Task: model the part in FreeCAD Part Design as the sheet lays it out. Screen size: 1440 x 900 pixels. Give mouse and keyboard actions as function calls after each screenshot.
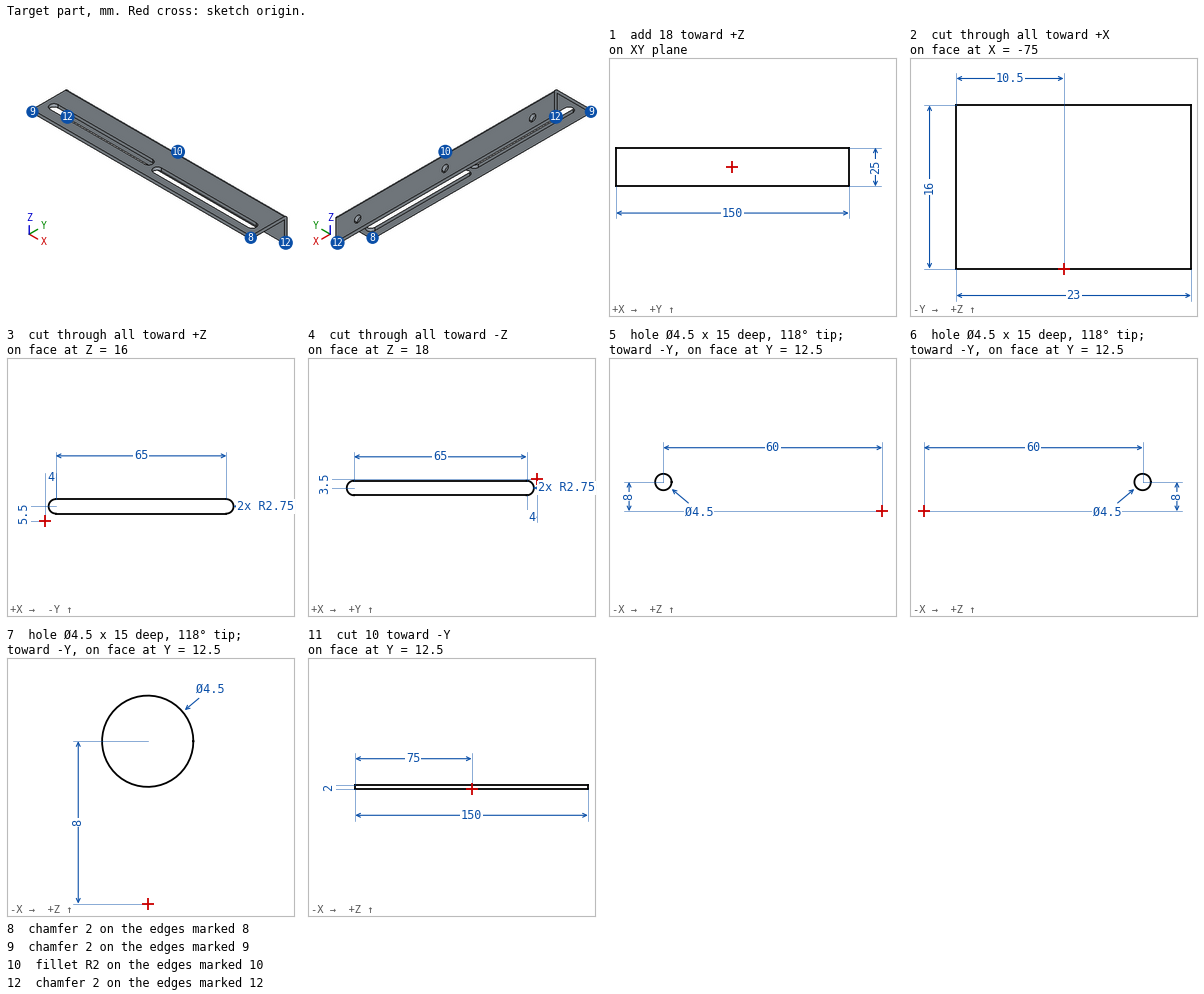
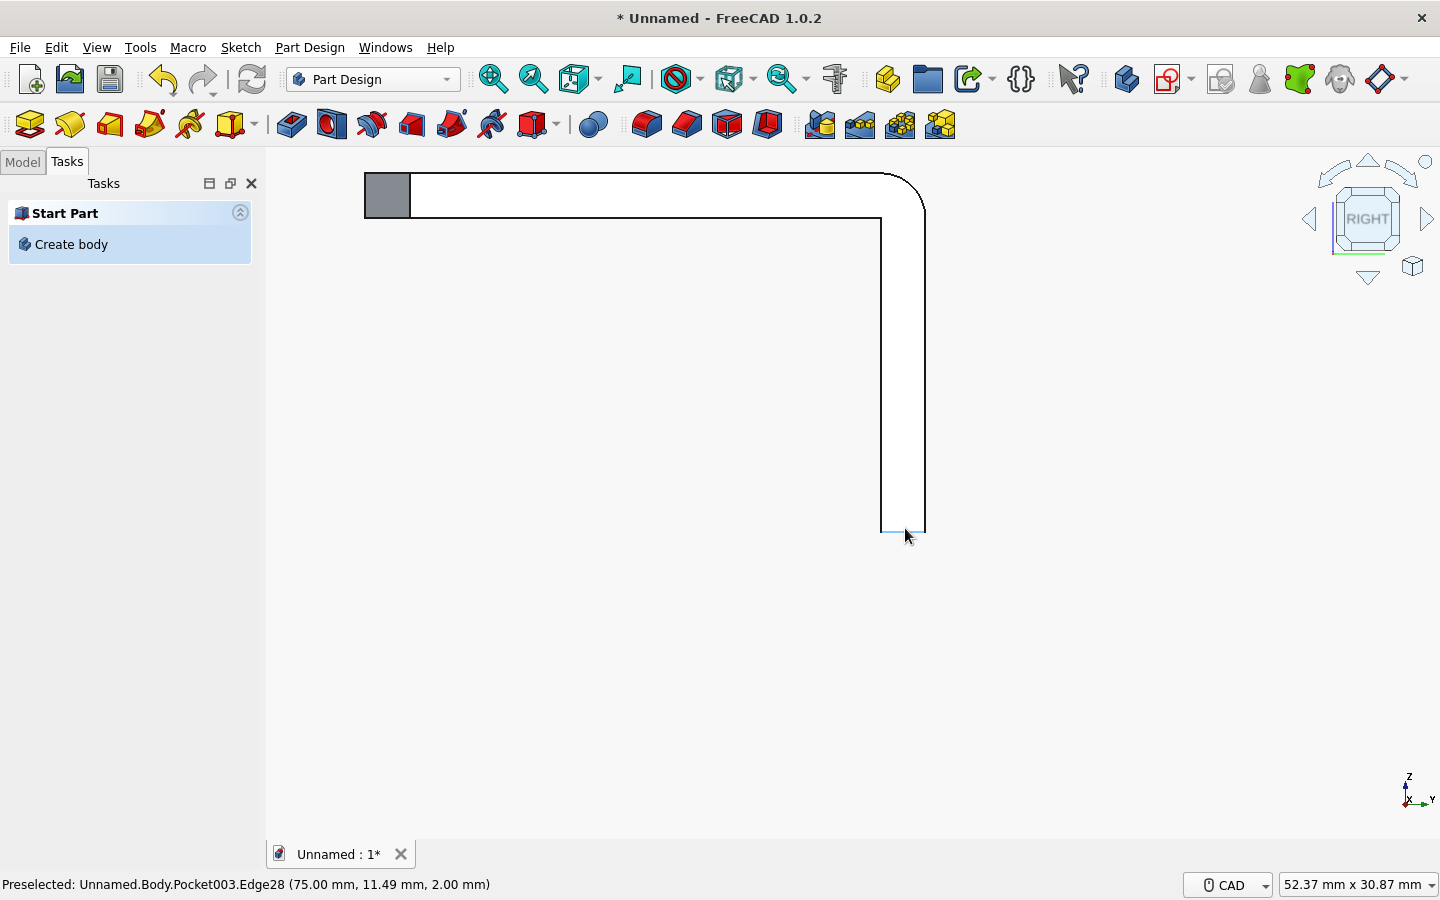
click(903, 531)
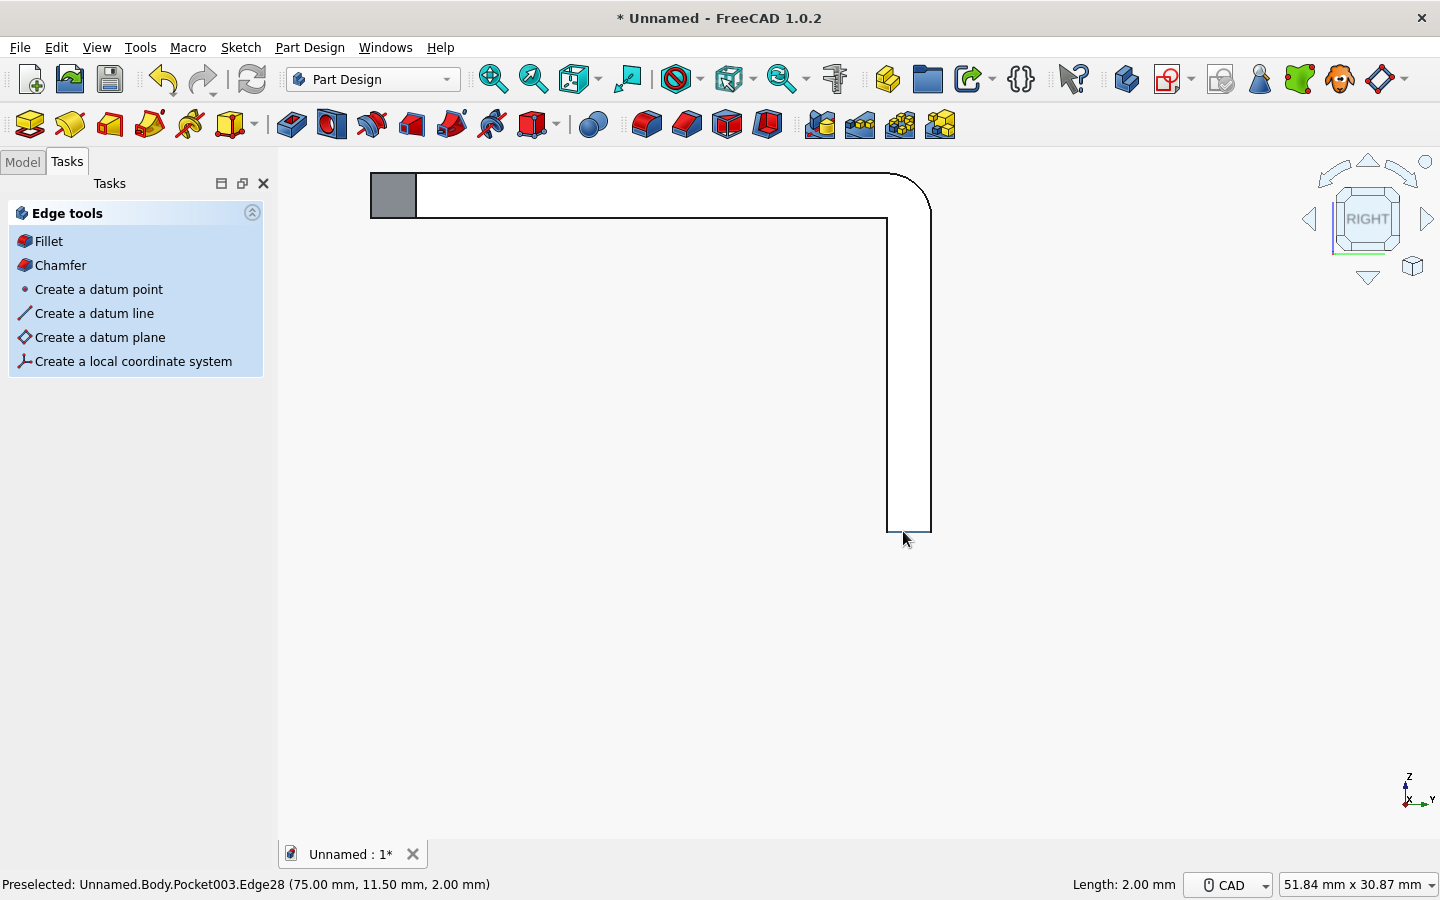
click(494, 80)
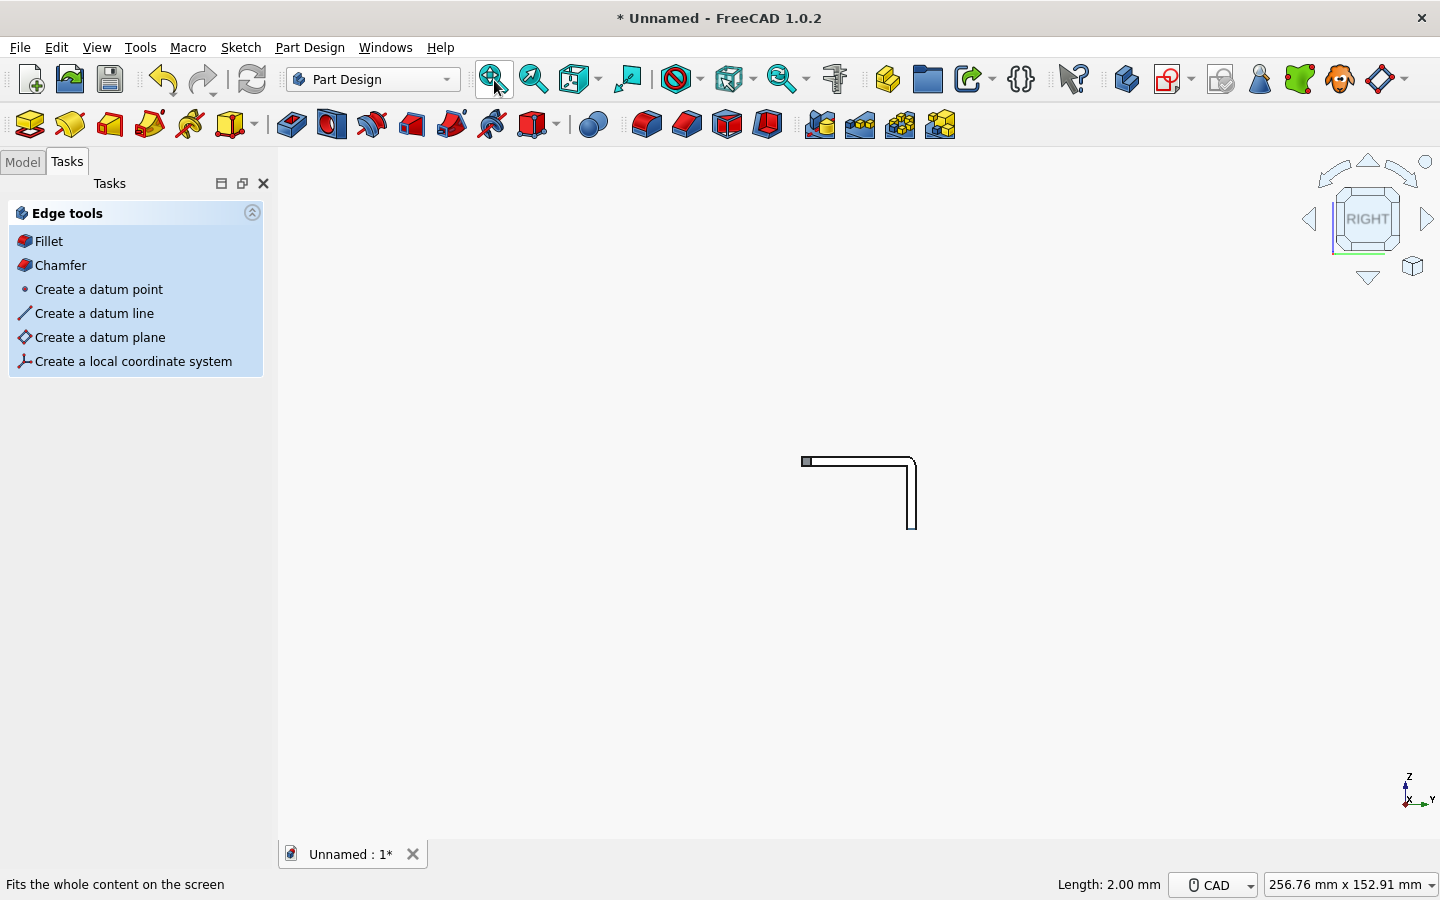
key(5)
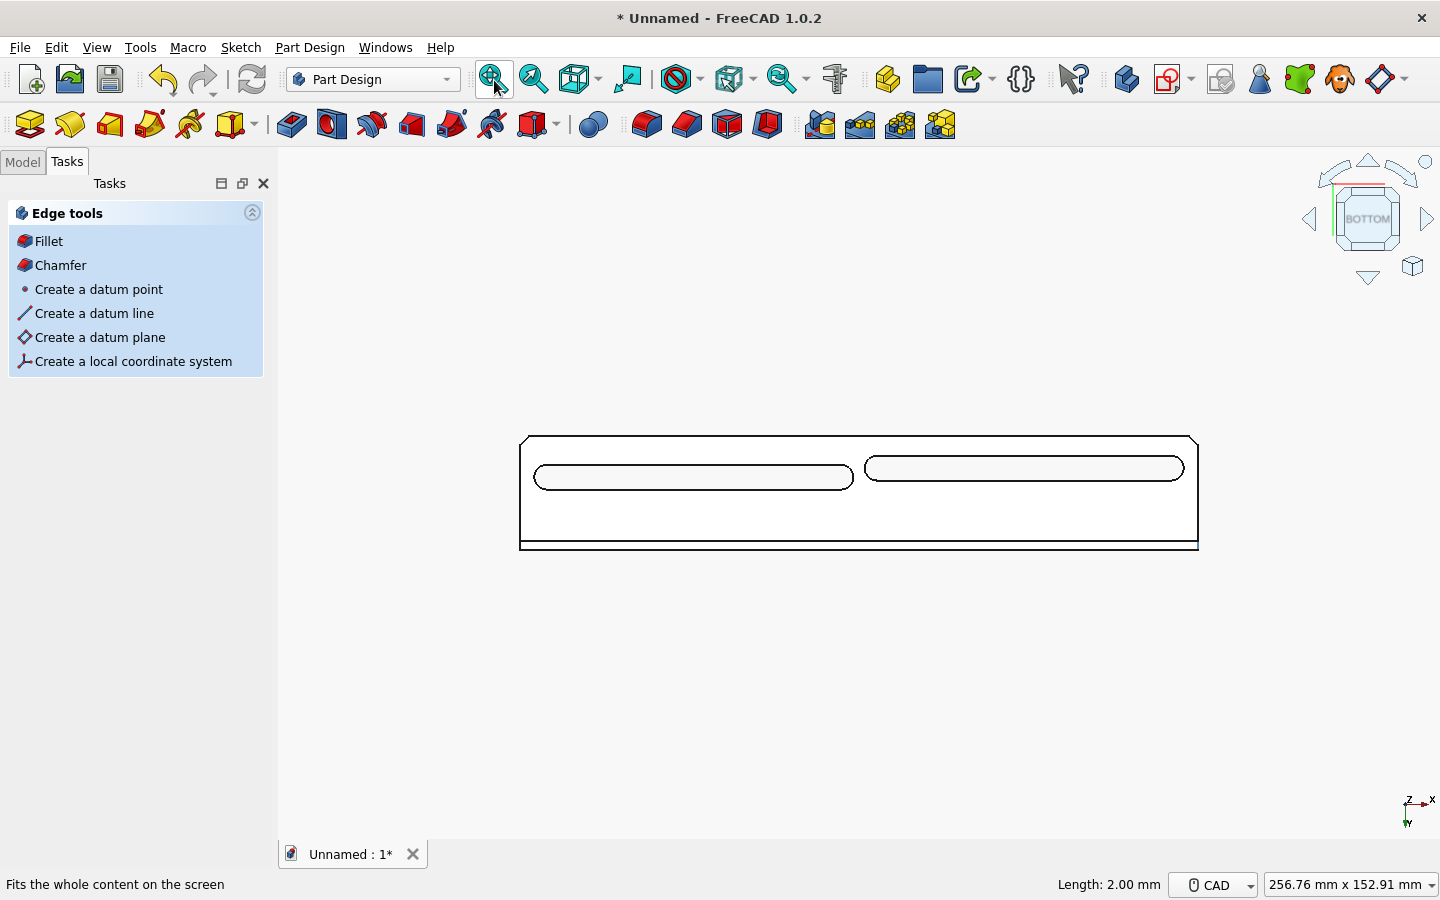
scroll(520, 544, up, 8)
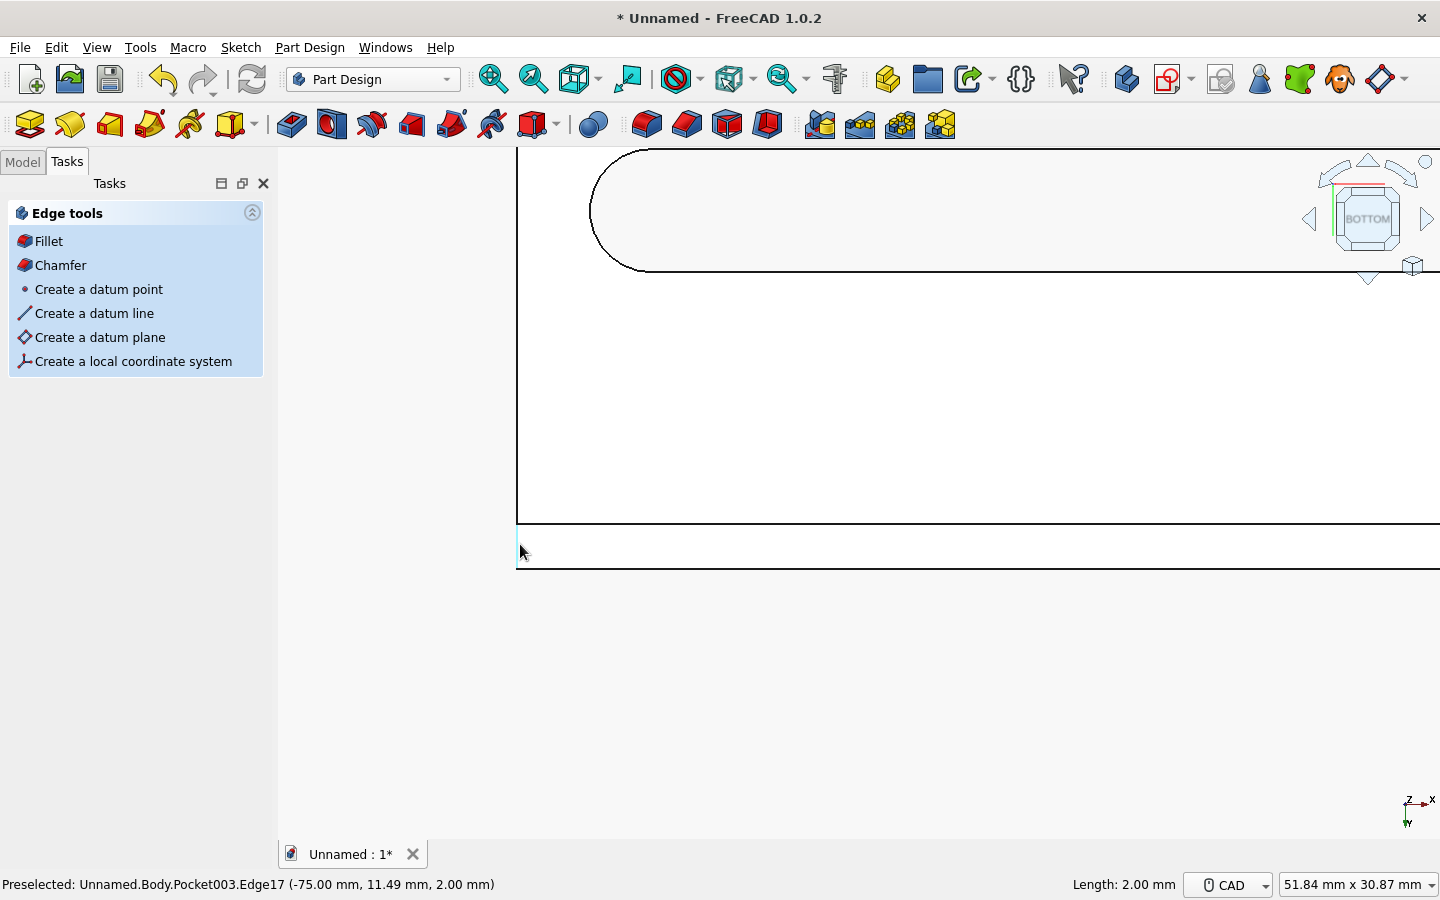
click(517, 546, ctrl)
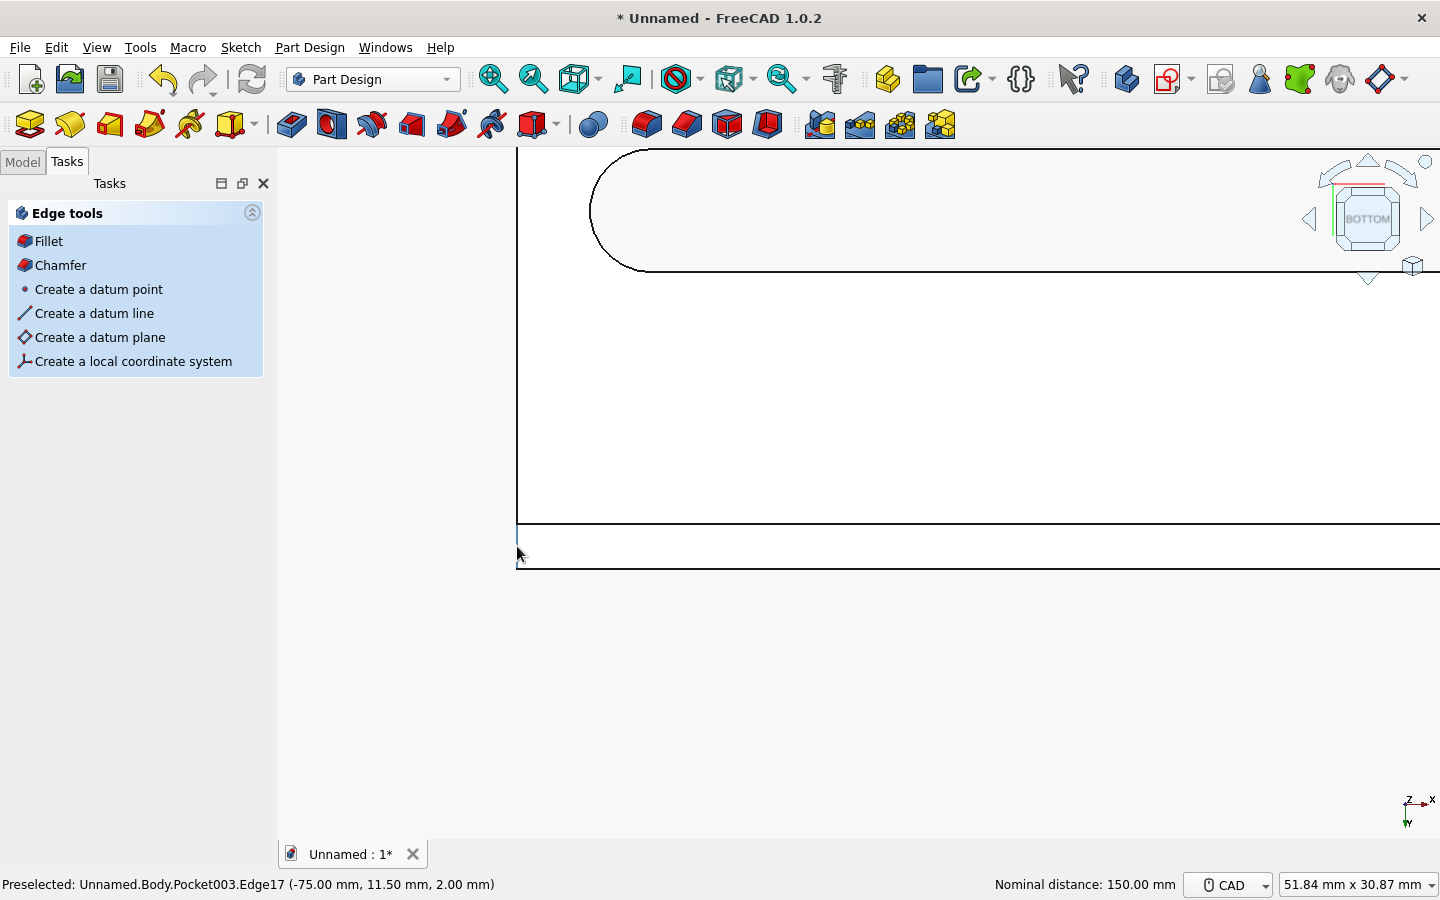
click(688, 124)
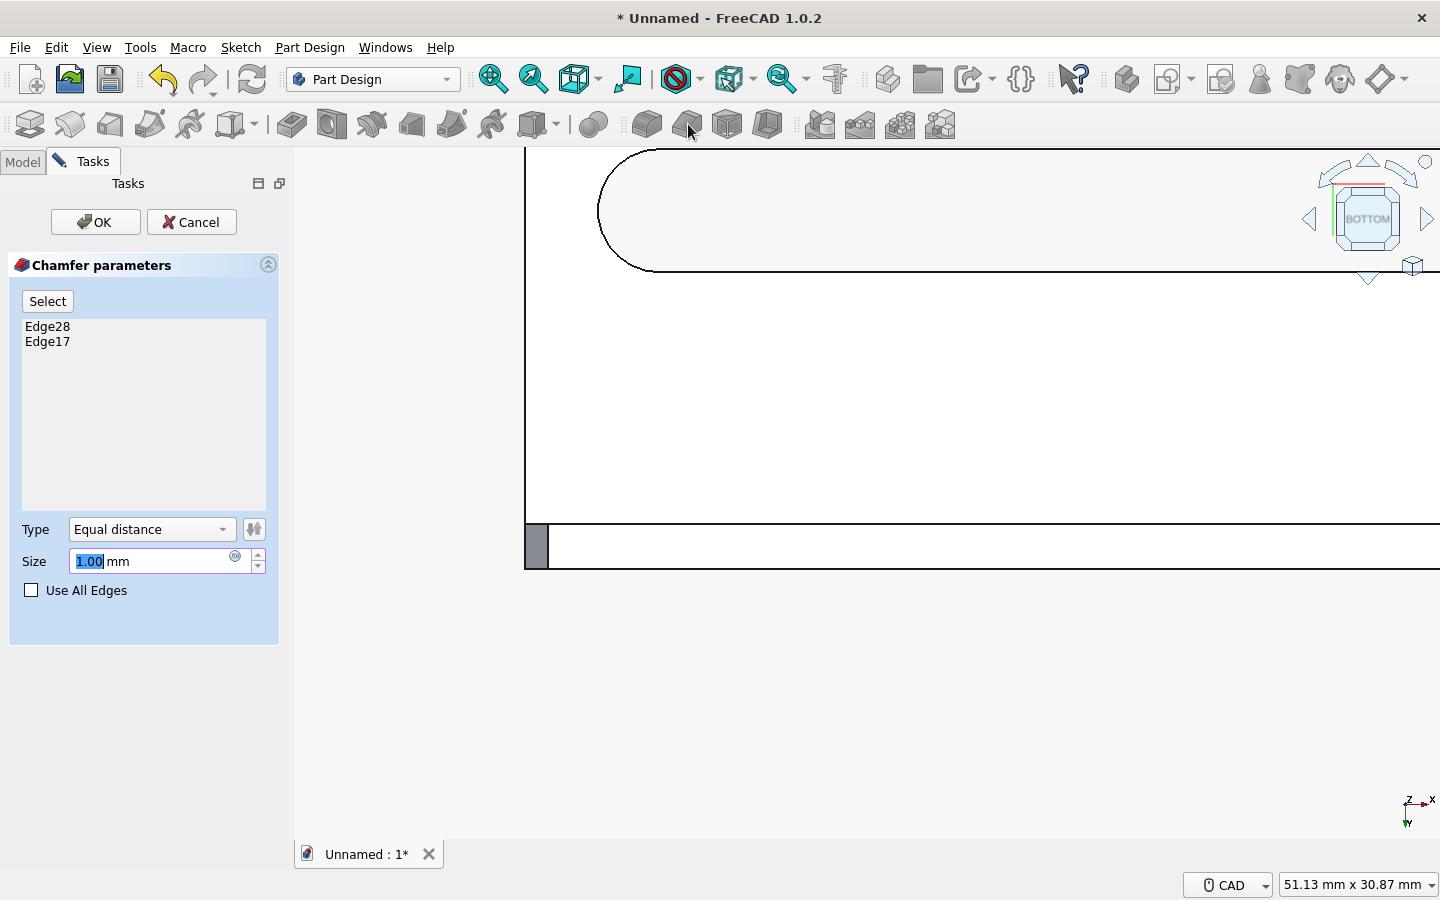
text(2)
key(Tab)